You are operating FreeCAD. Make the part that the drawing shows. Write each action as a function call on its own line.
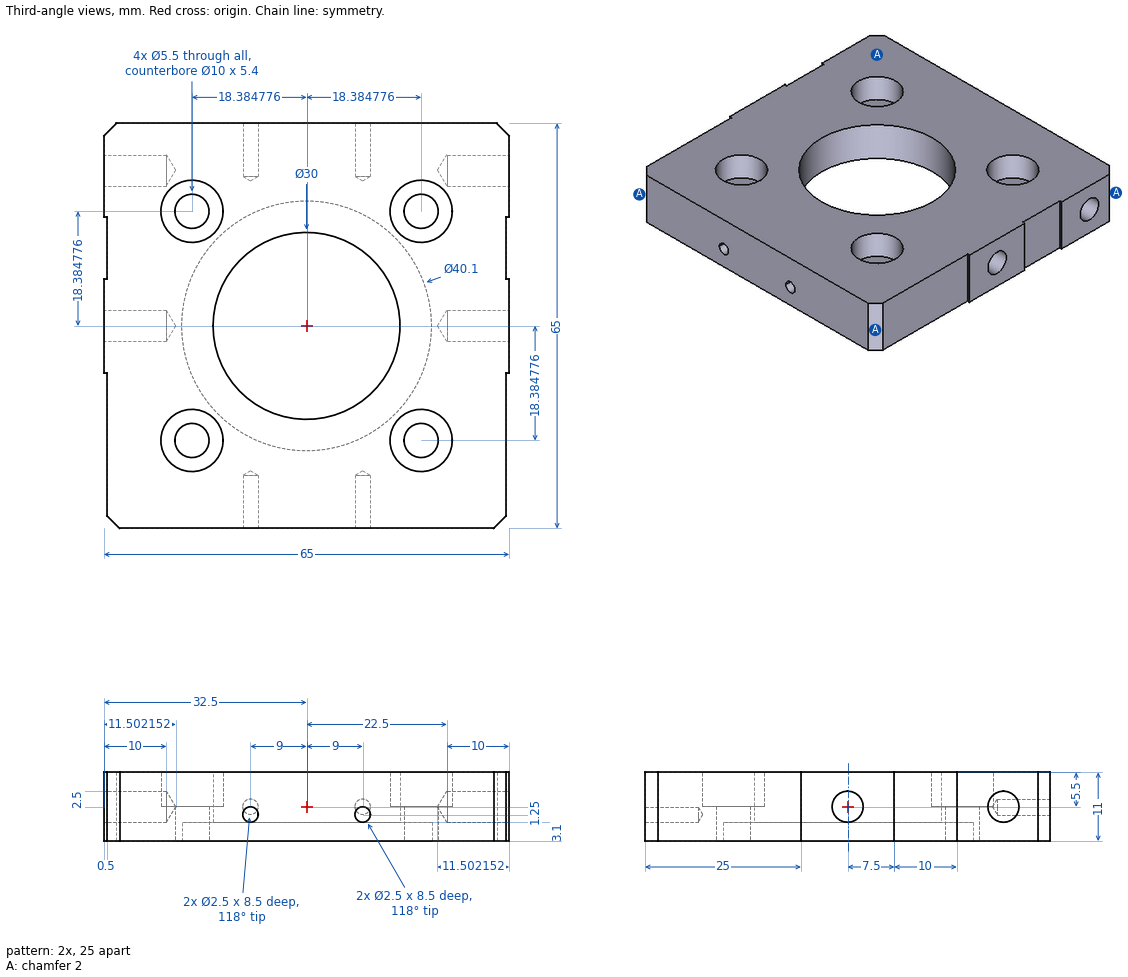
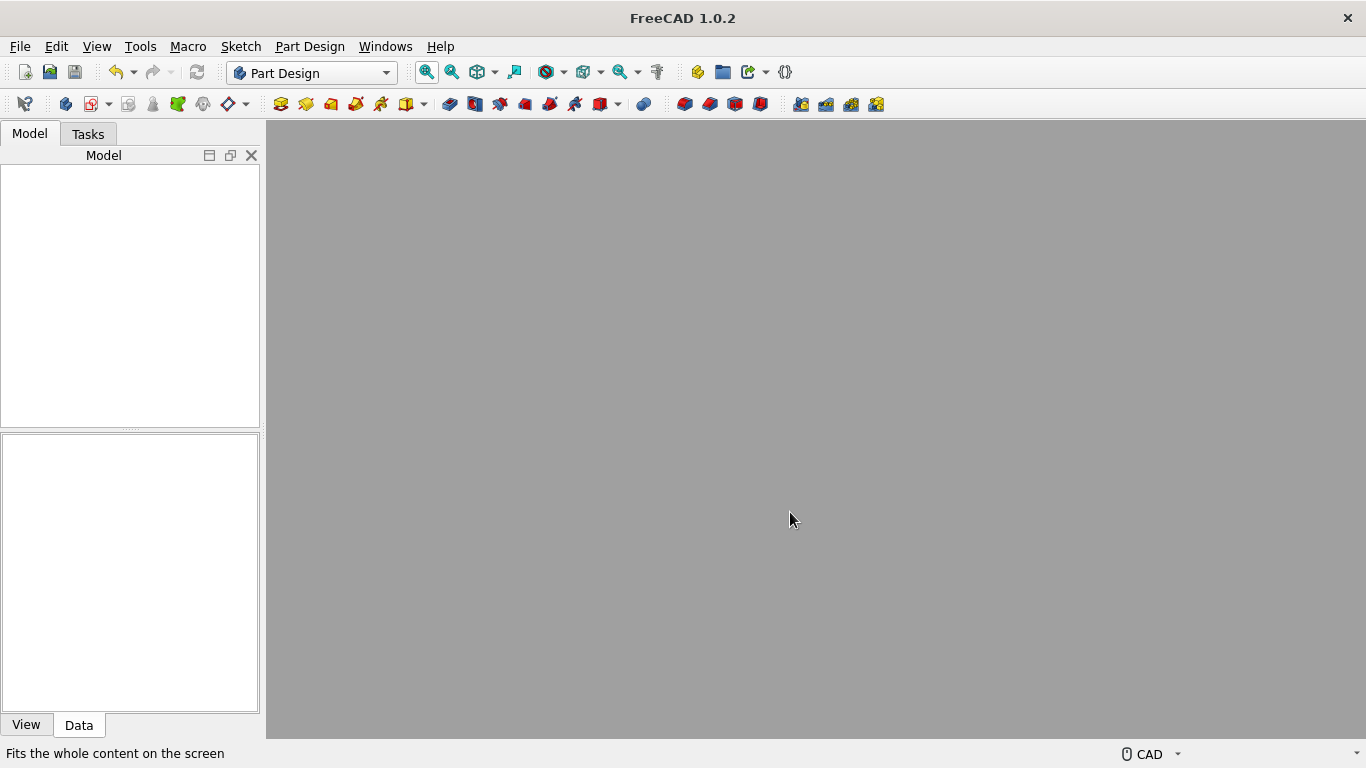
click(25, 72)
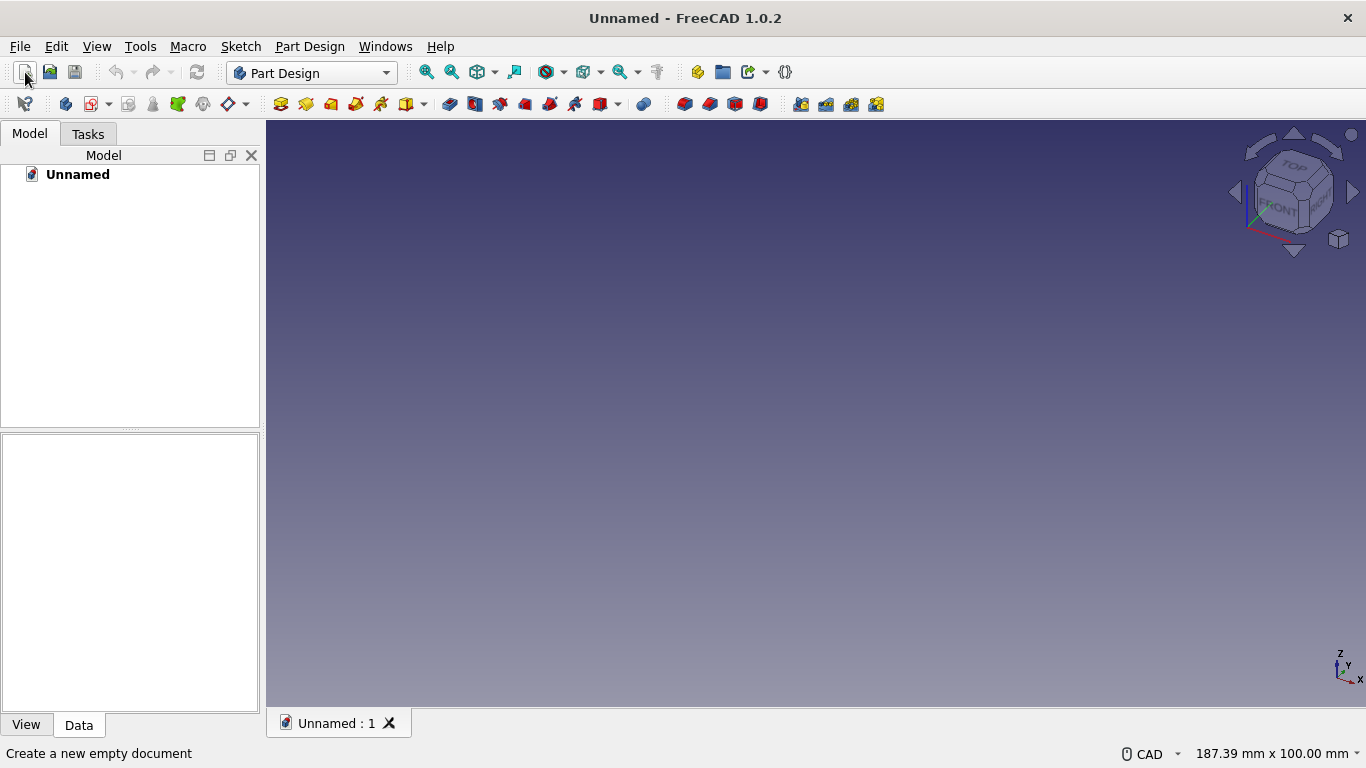
click(90, 104)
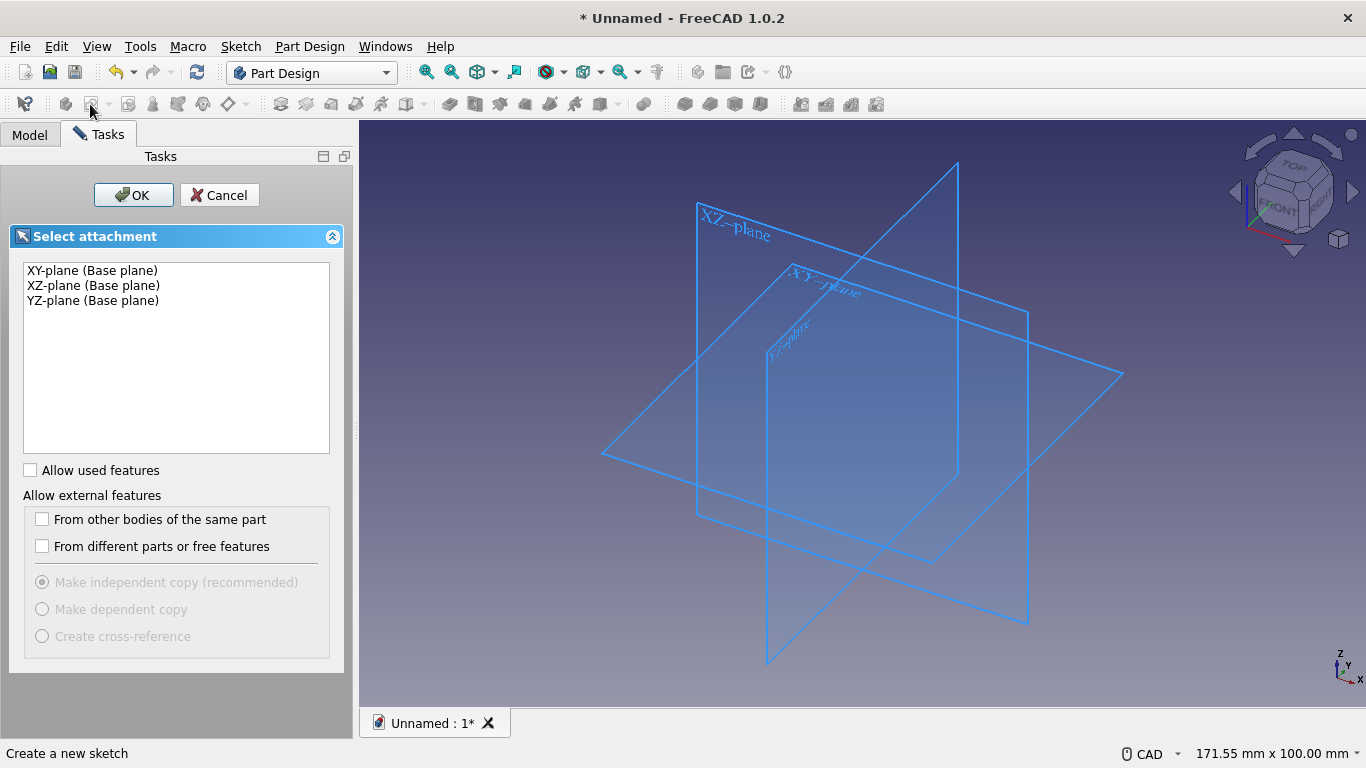
click(84, 270)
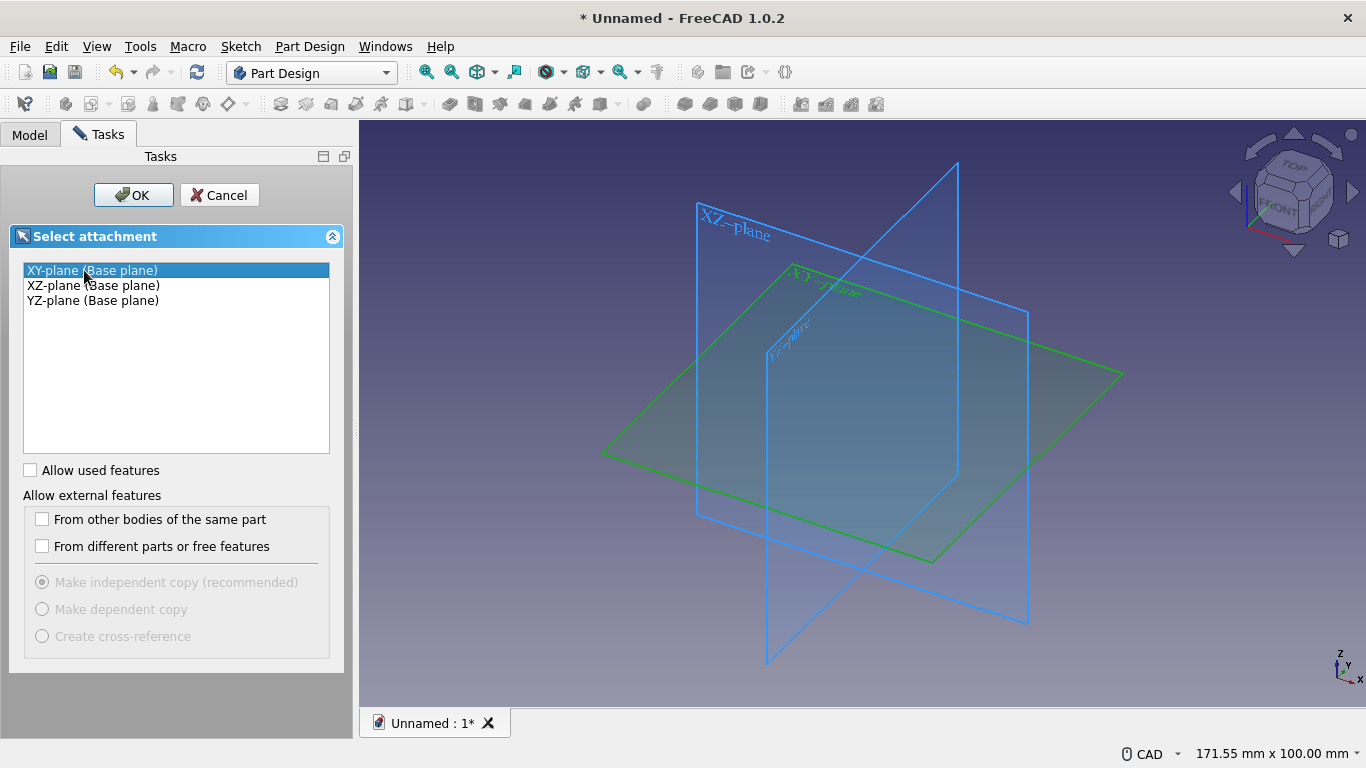
click(134, 195)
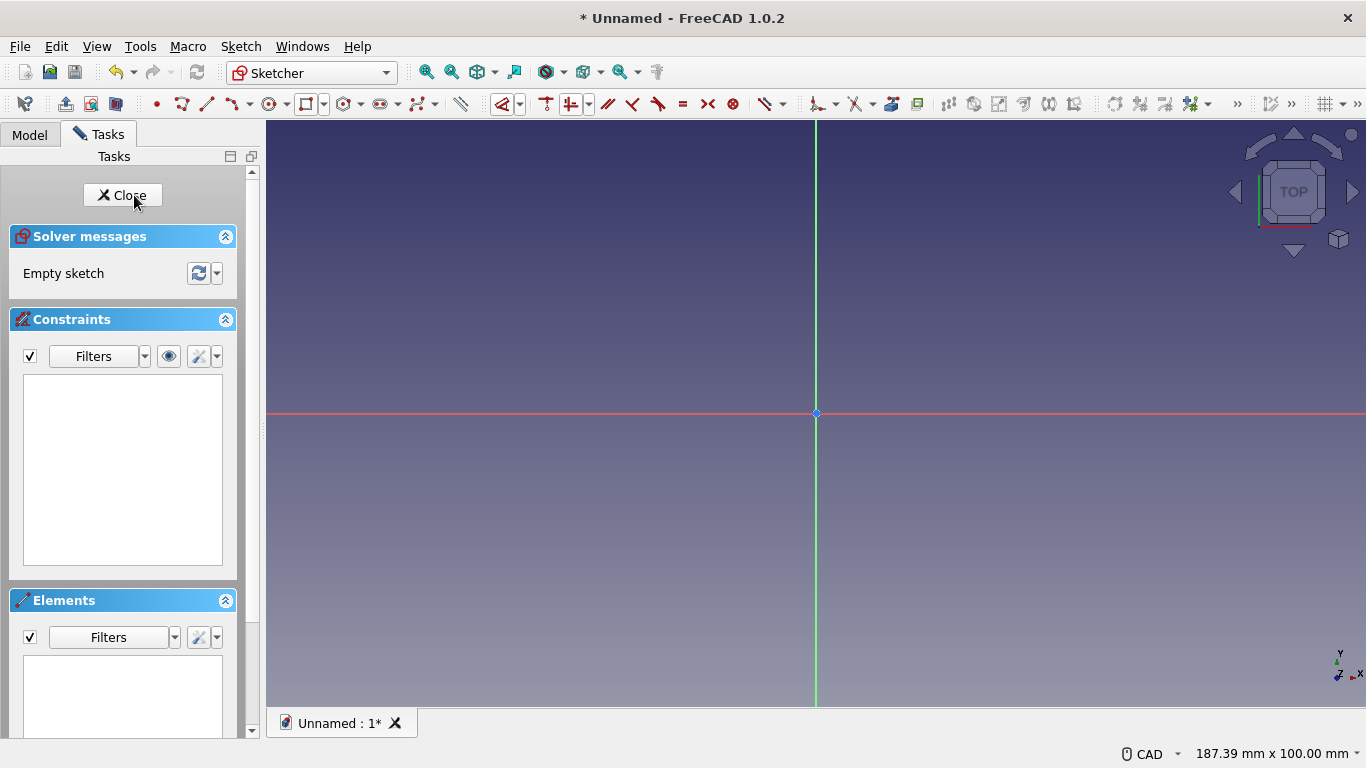
click(324, 104)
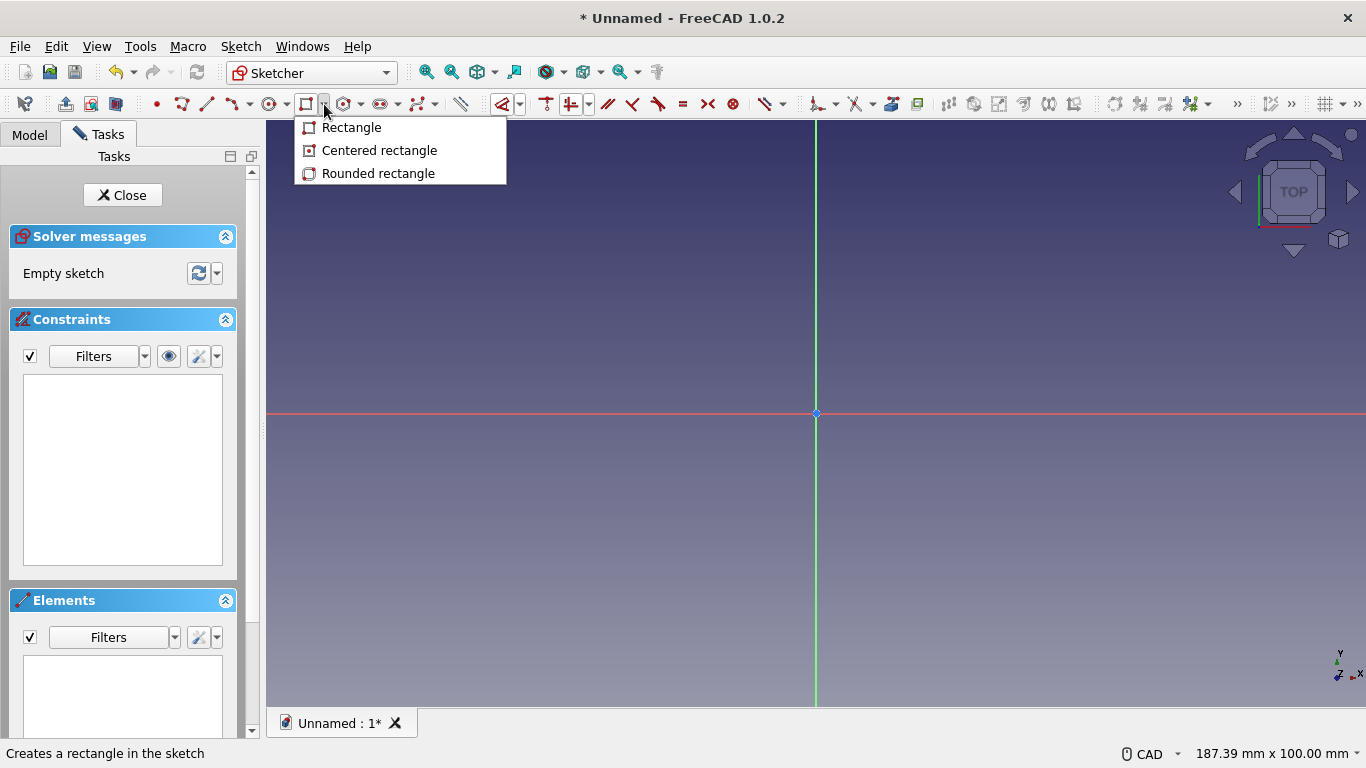
click(400, 150)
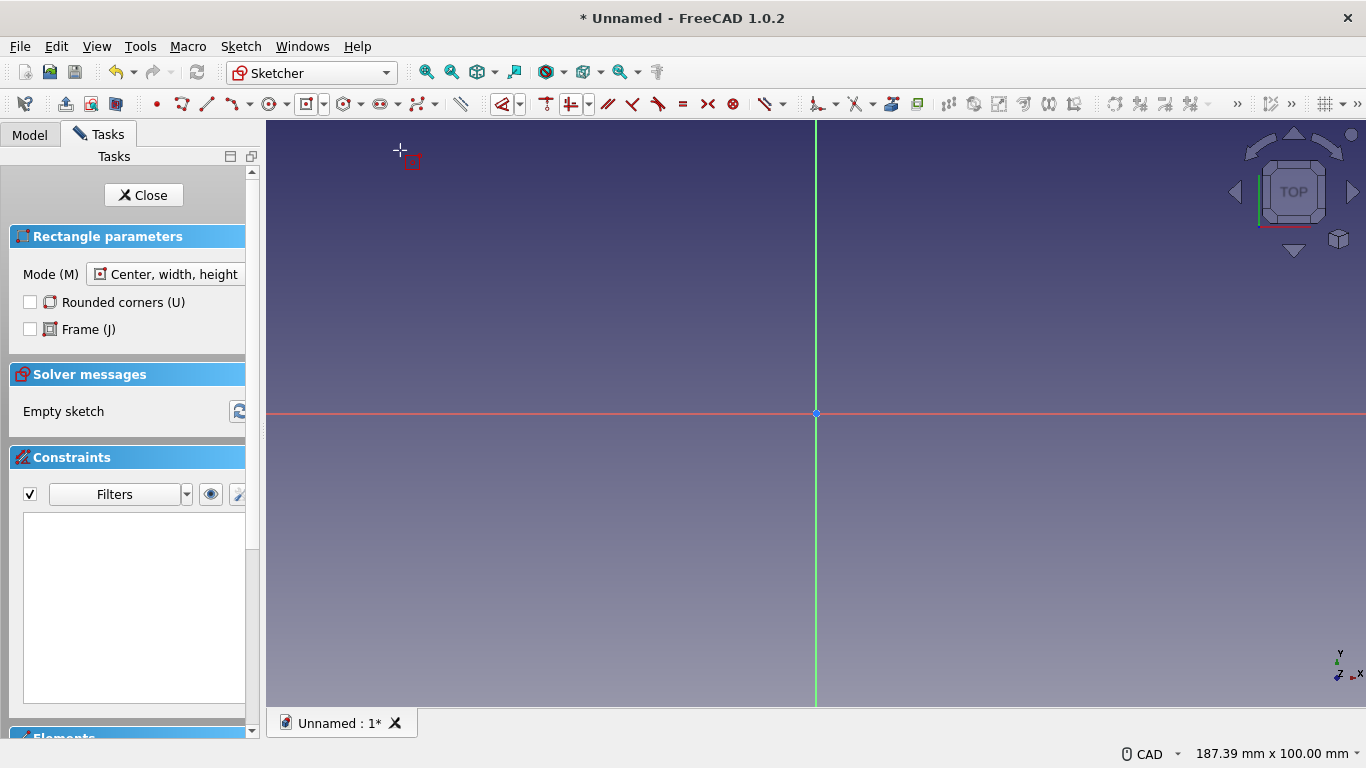
click(816, 414)
click(1007, 223)
key(Escape)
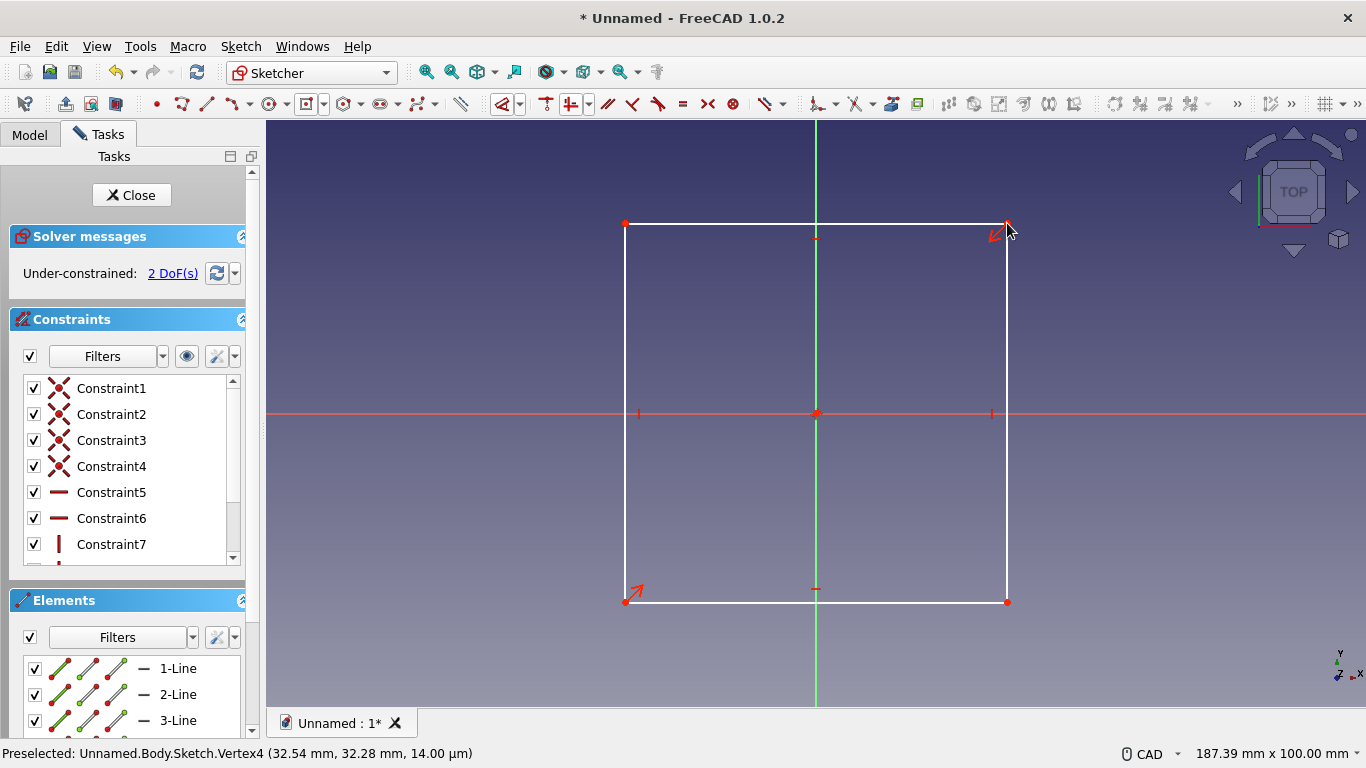
click(740, 603)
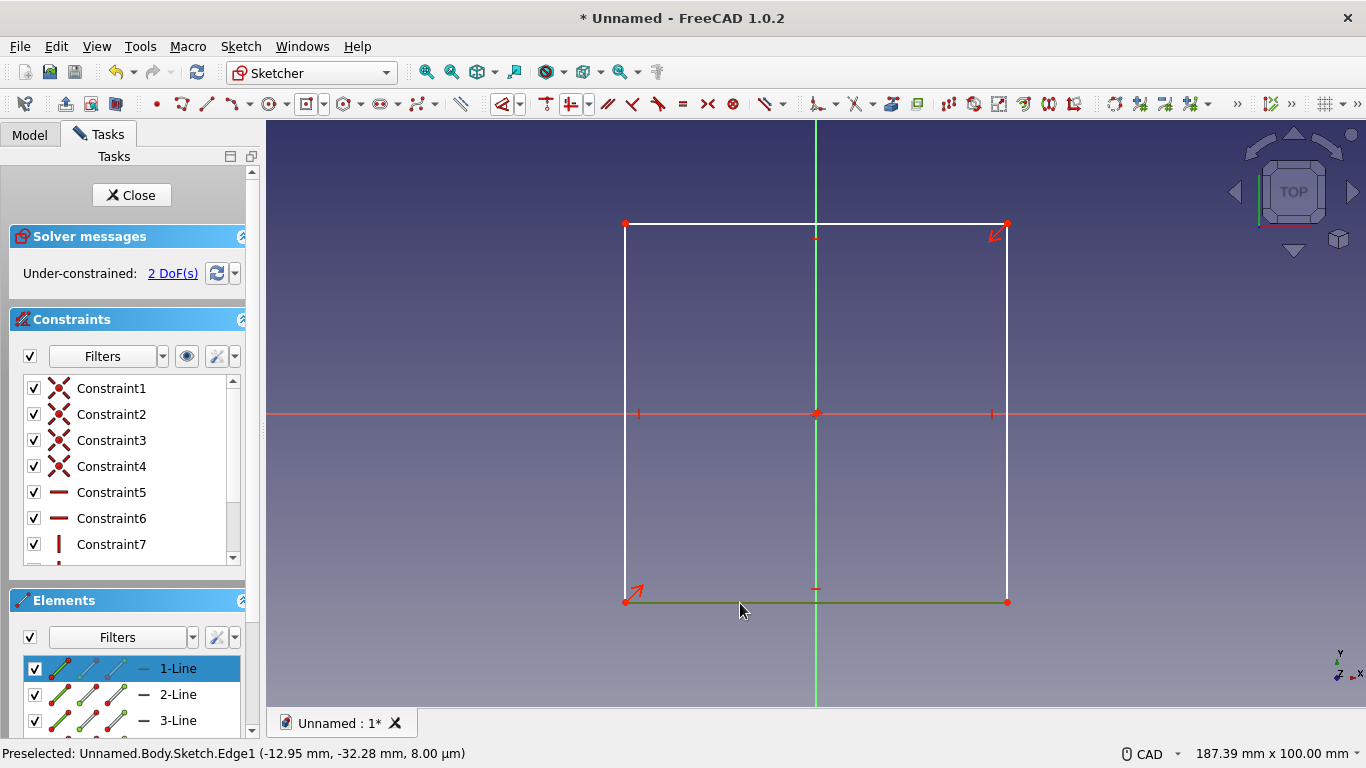
click(520, 104)